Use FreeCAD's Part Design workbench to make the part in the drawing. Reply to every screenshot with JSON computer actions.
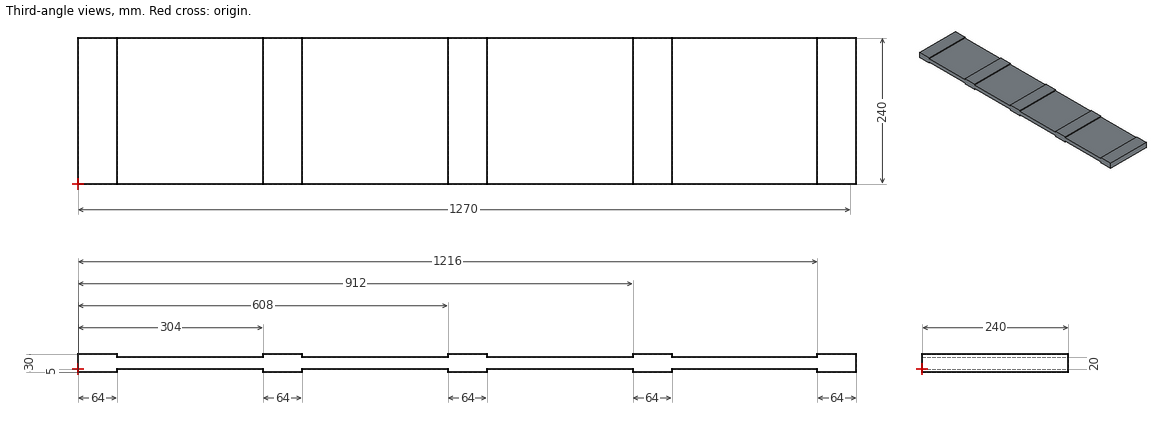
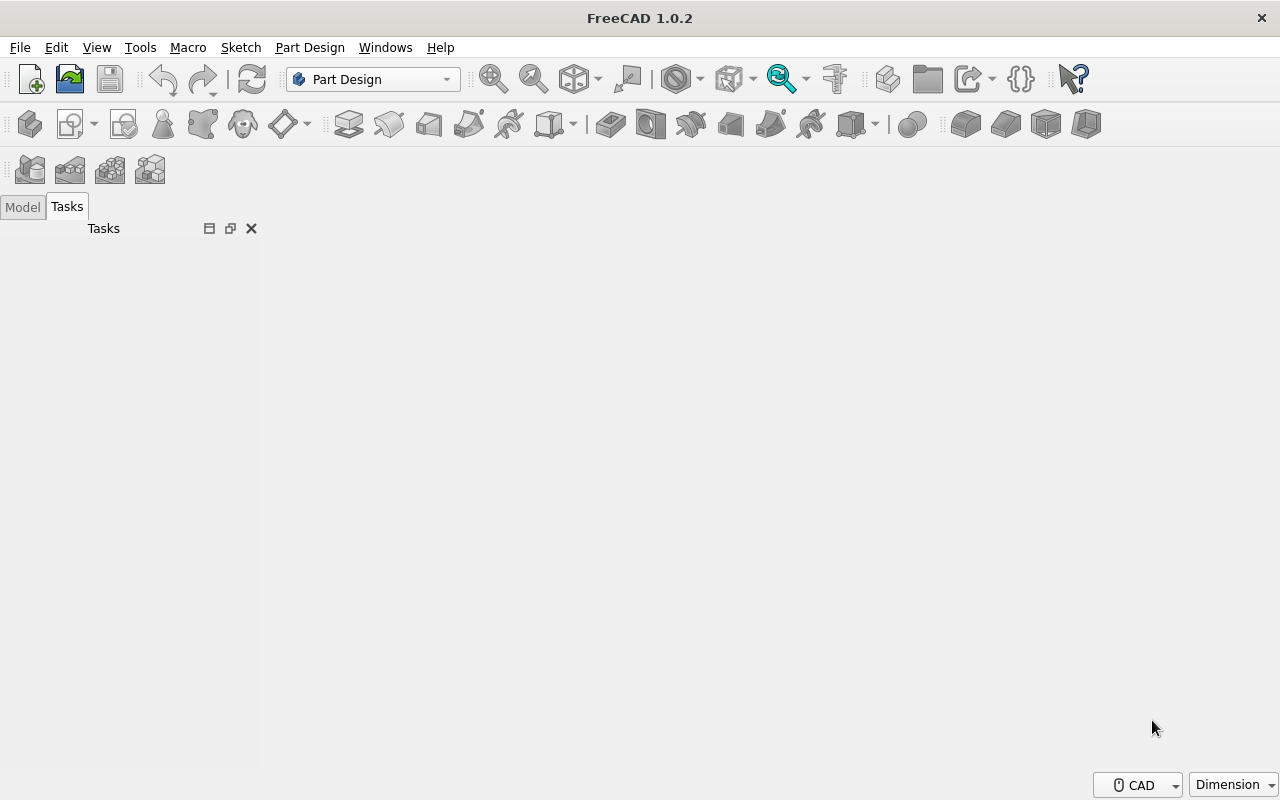
{"action": "left_click", "coordinate": [30, 80]}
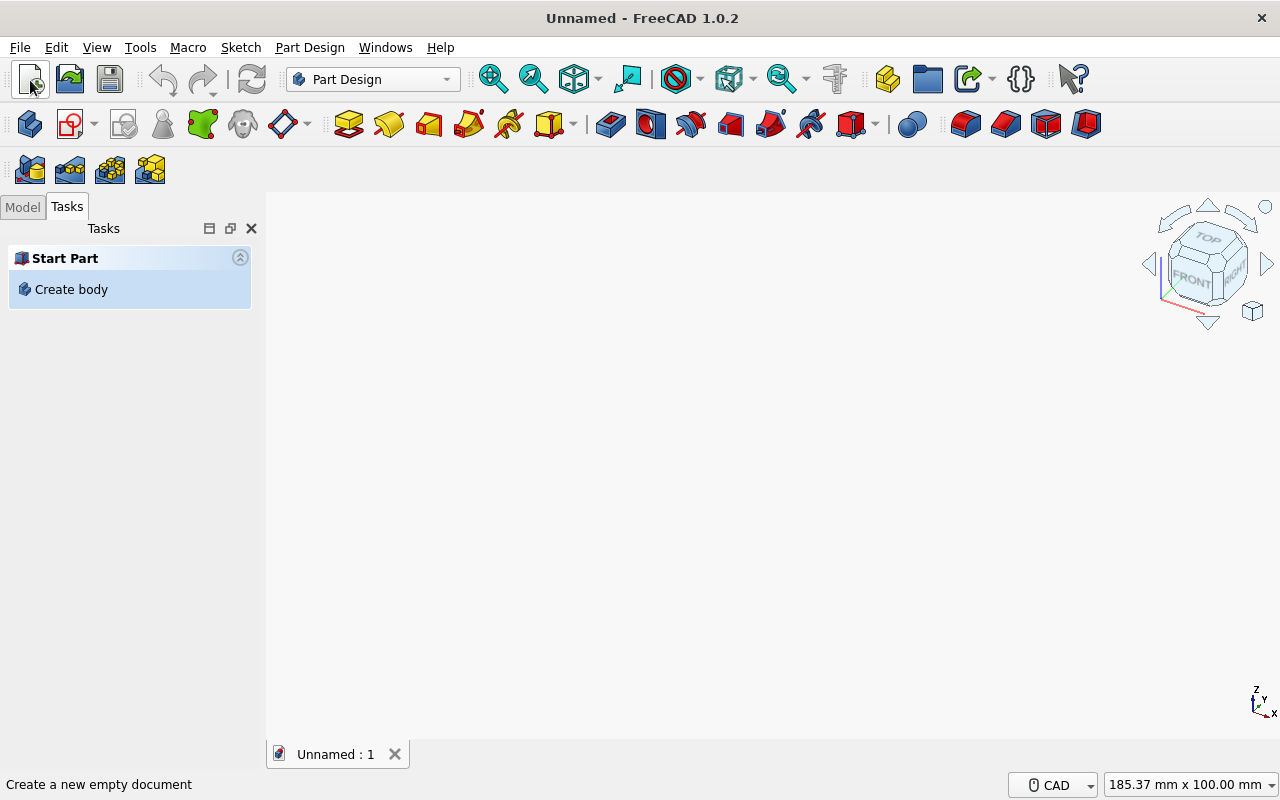
{"action": "left_click", "coordinate": [70, 124]}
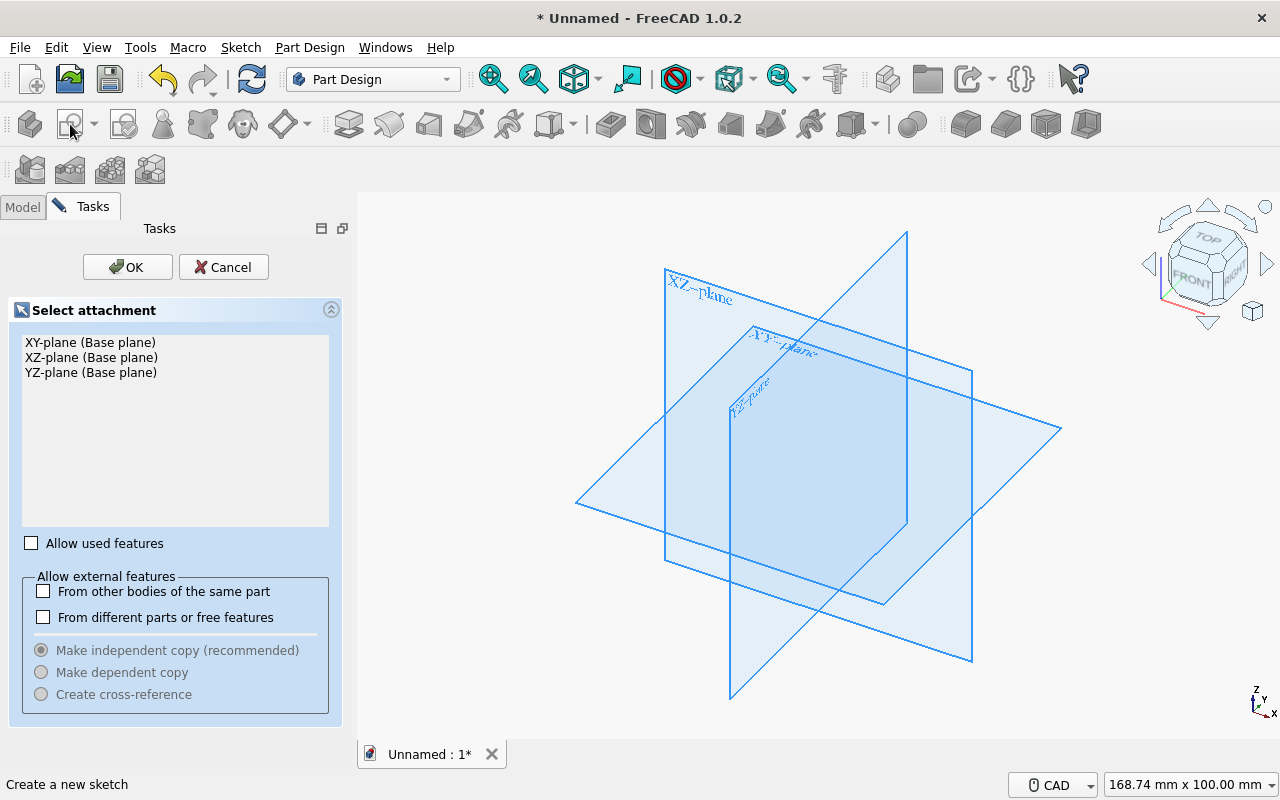
{"action": "left_click", "coordinate": [82, 342]}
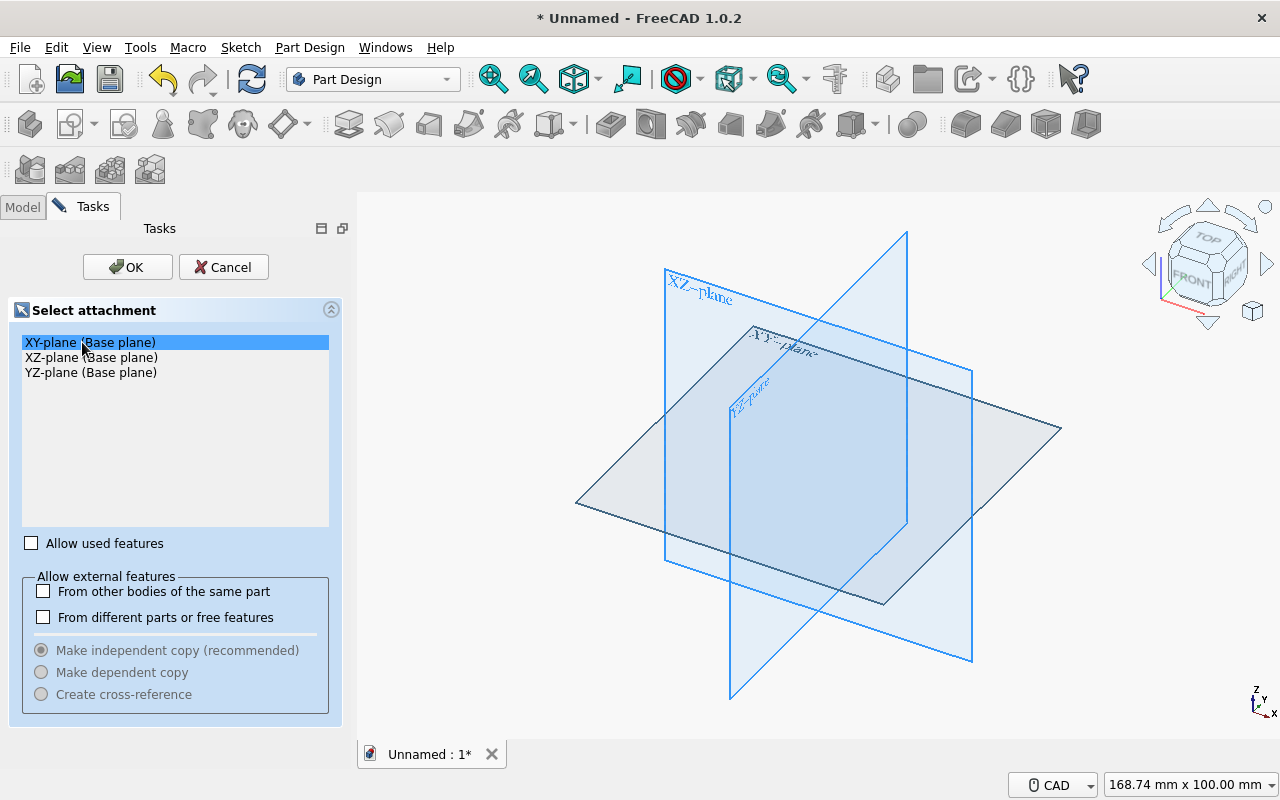
{"action": "left_click", "coordinate": [128, 267]}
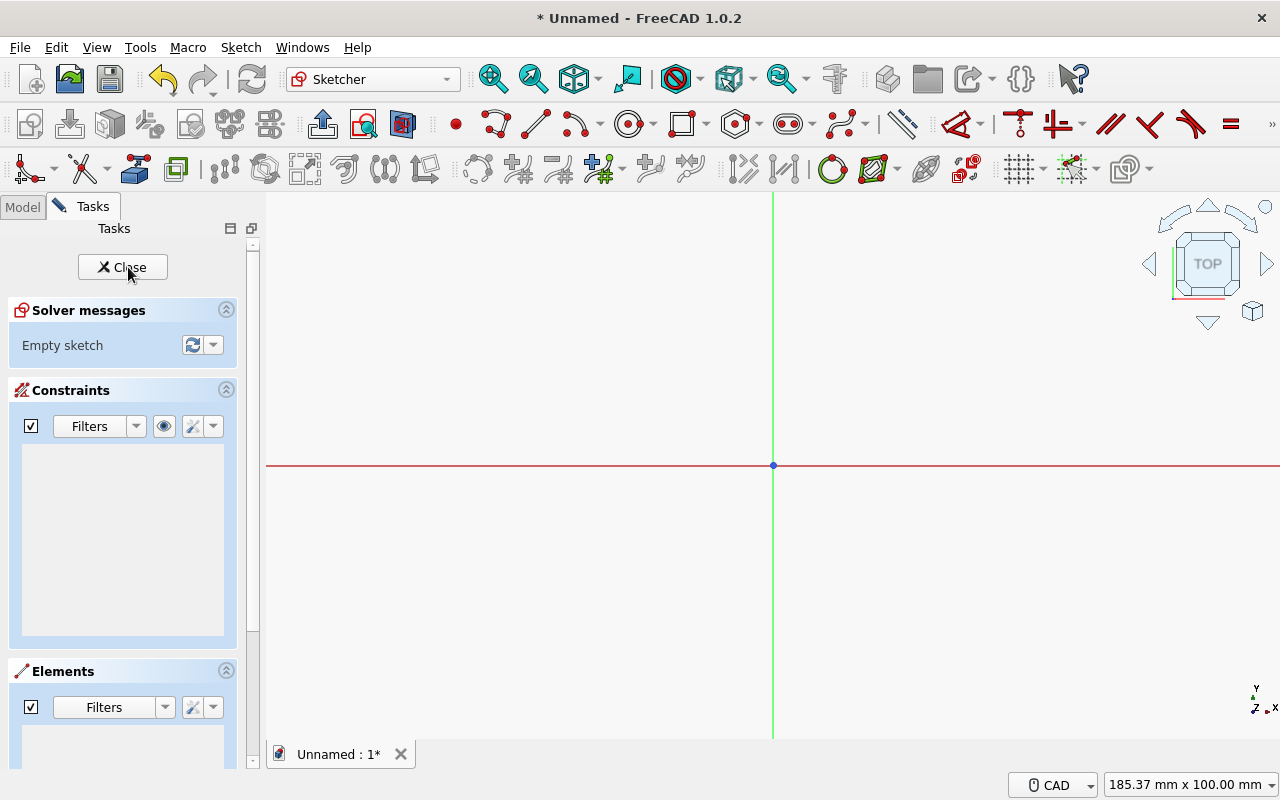
{"action": "scroll", "coordinate": [351, 531], "scroll_direction": "down", "scroll_amount": 12}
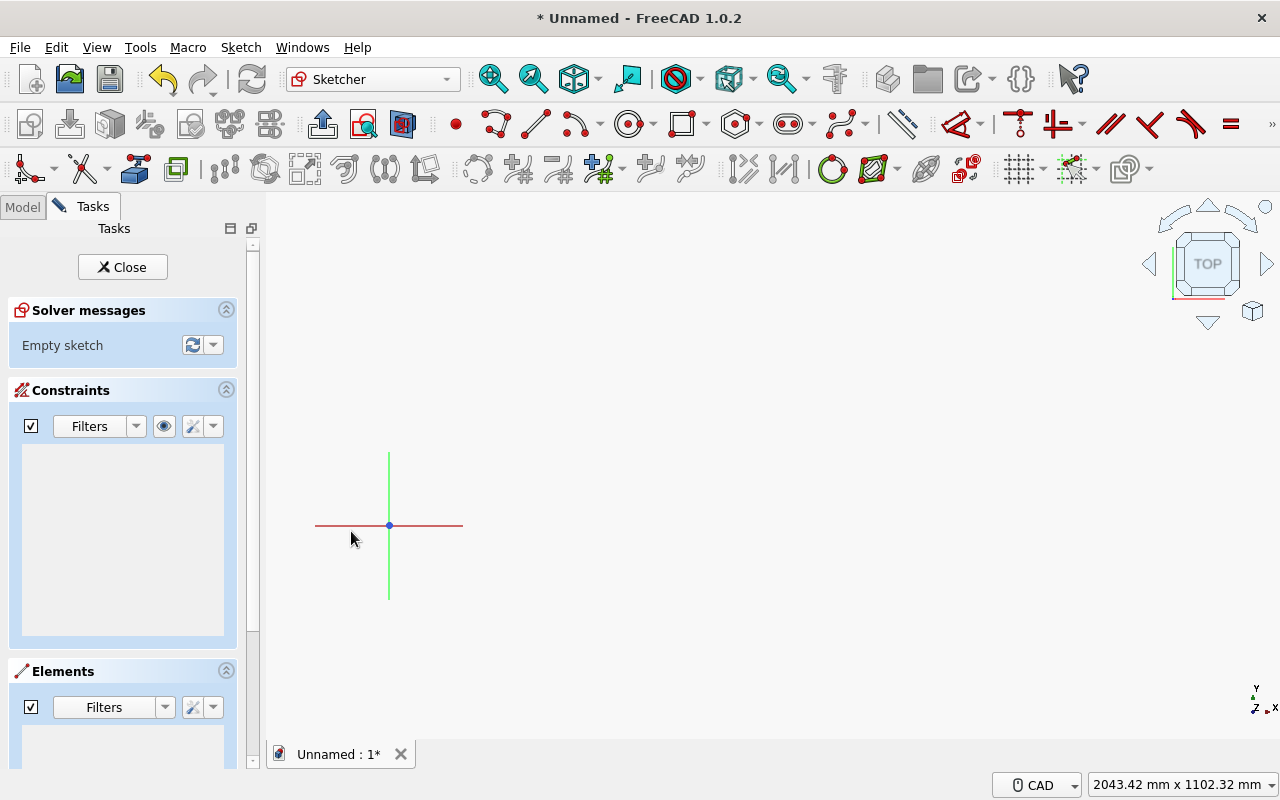
{"action": "key", "text": "g r"}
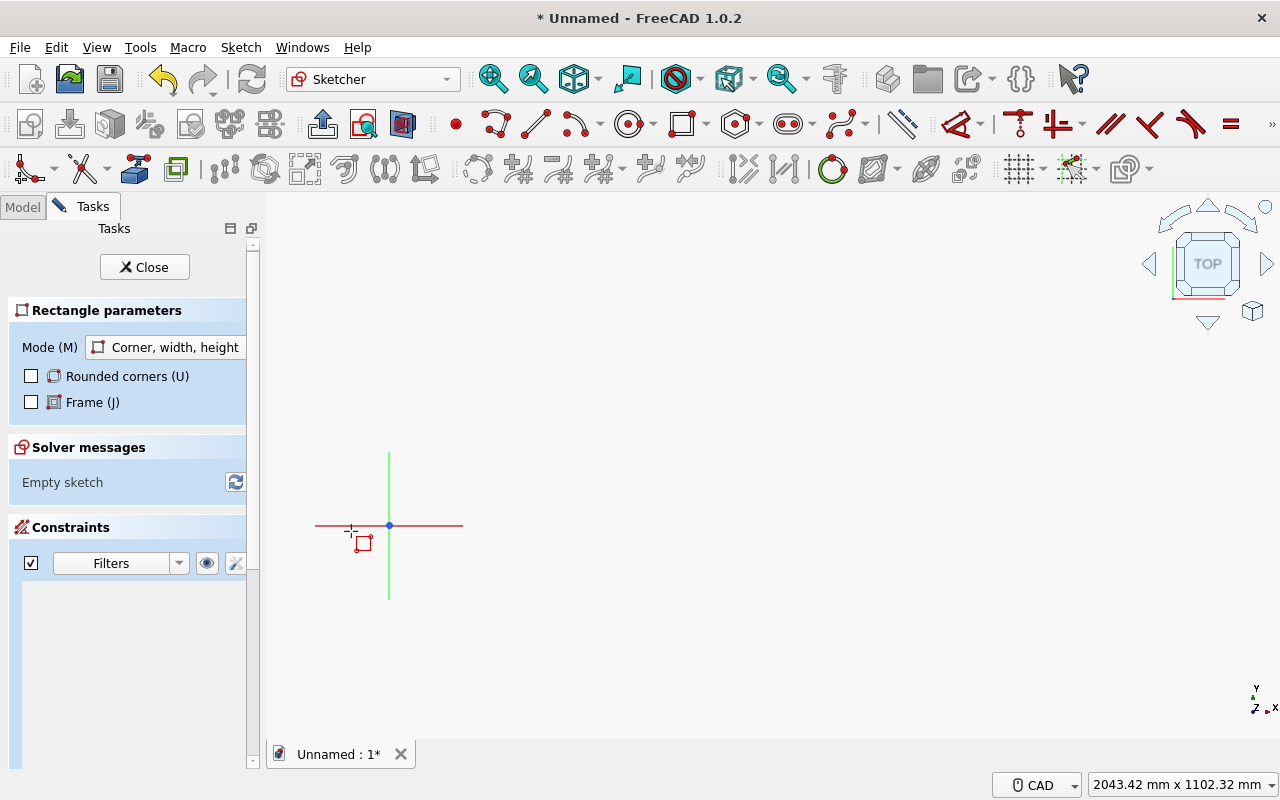
{"action": "left_click", "coordinate": [389, 526]}
{"action": "mouse_move", "coordinate": [1020, 407]}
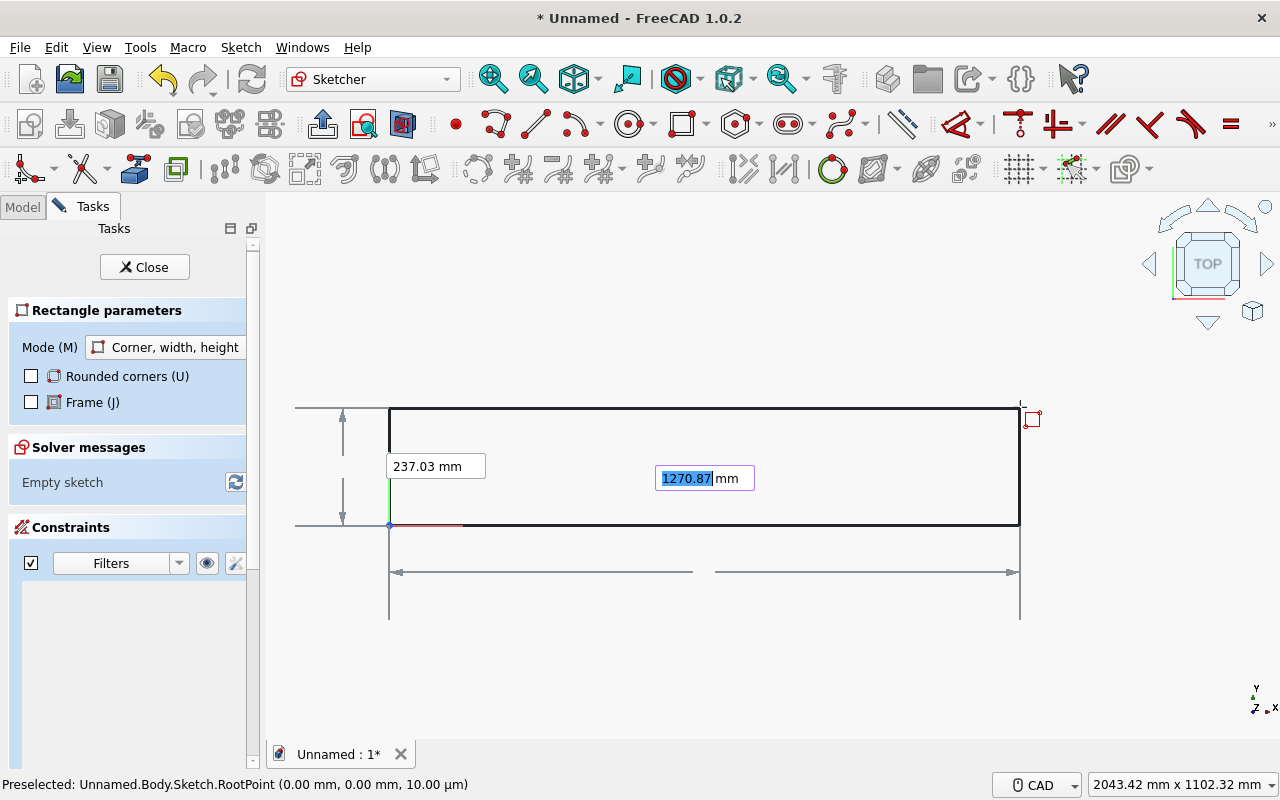
{"action": "type", "text": "1270"}
{"action": "key", "text": "Tab"}
{"action": "type", "text": "240"}
{"action": "key", "text": "Return"}
{"action": "key", "text": "Escape"}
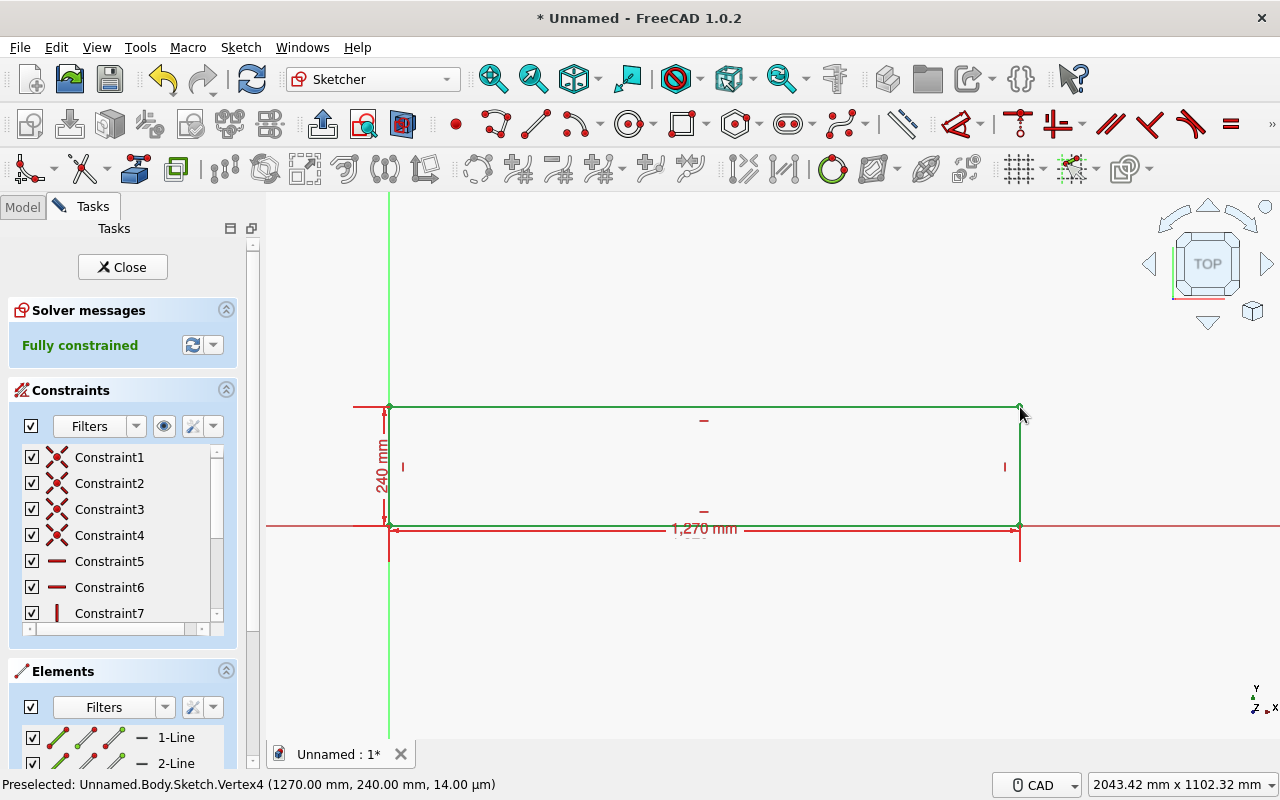
{"action": "left_click", "coordinate": [123, 267]}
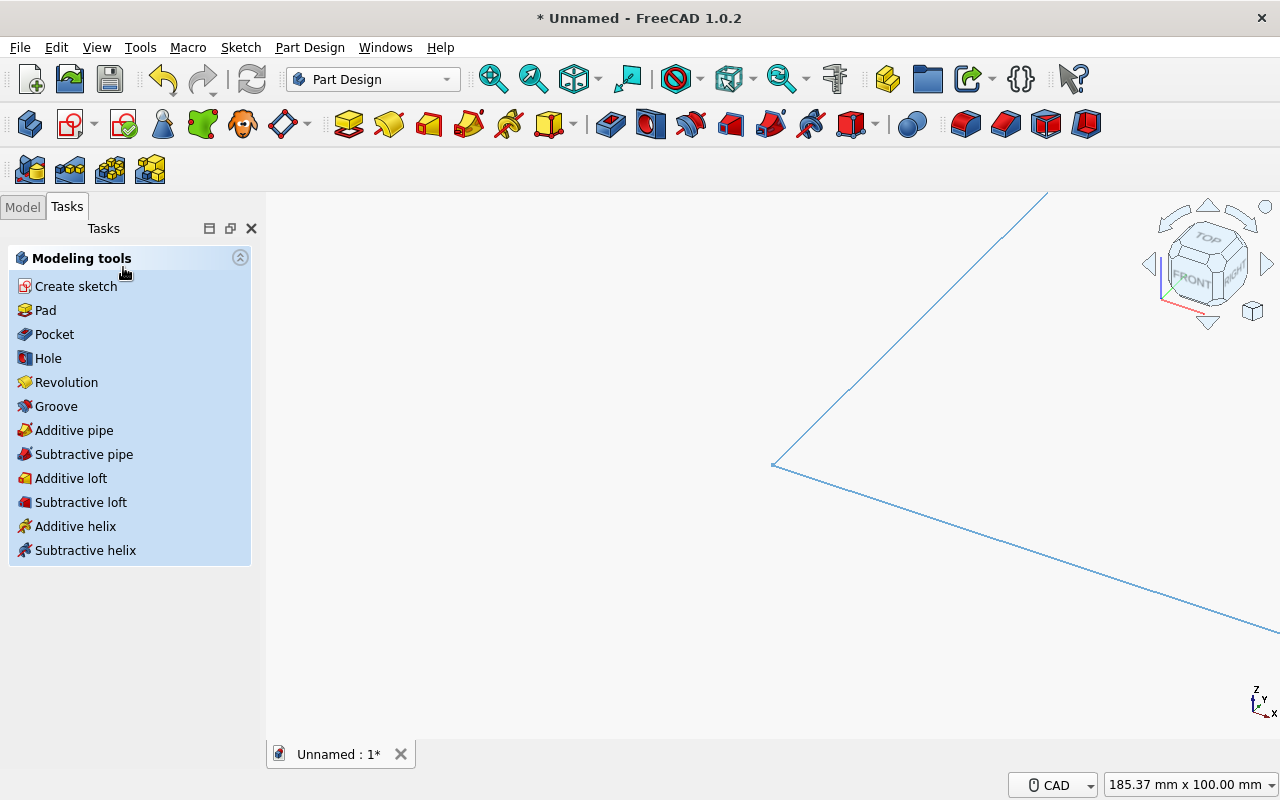
{"action": "left_click", "coordinate": [350, 124]}